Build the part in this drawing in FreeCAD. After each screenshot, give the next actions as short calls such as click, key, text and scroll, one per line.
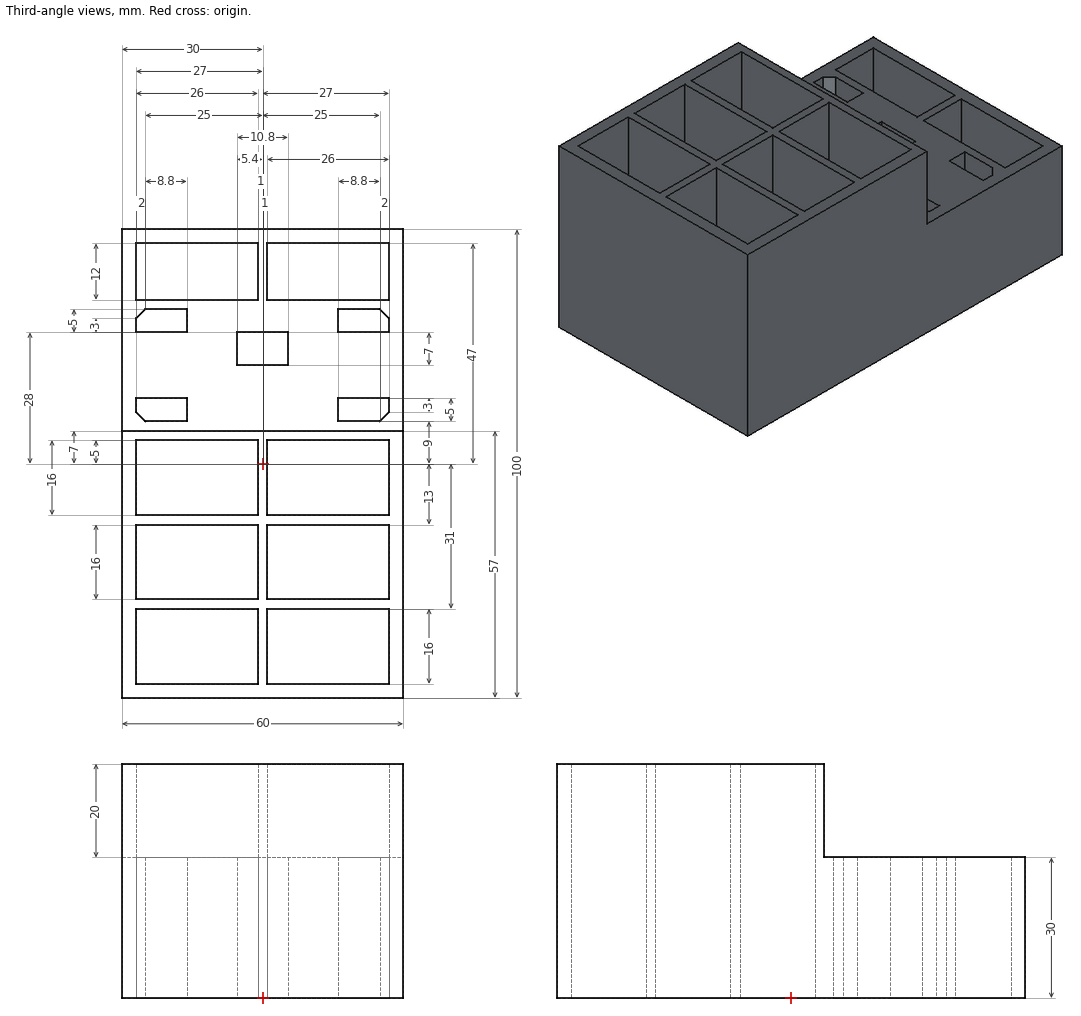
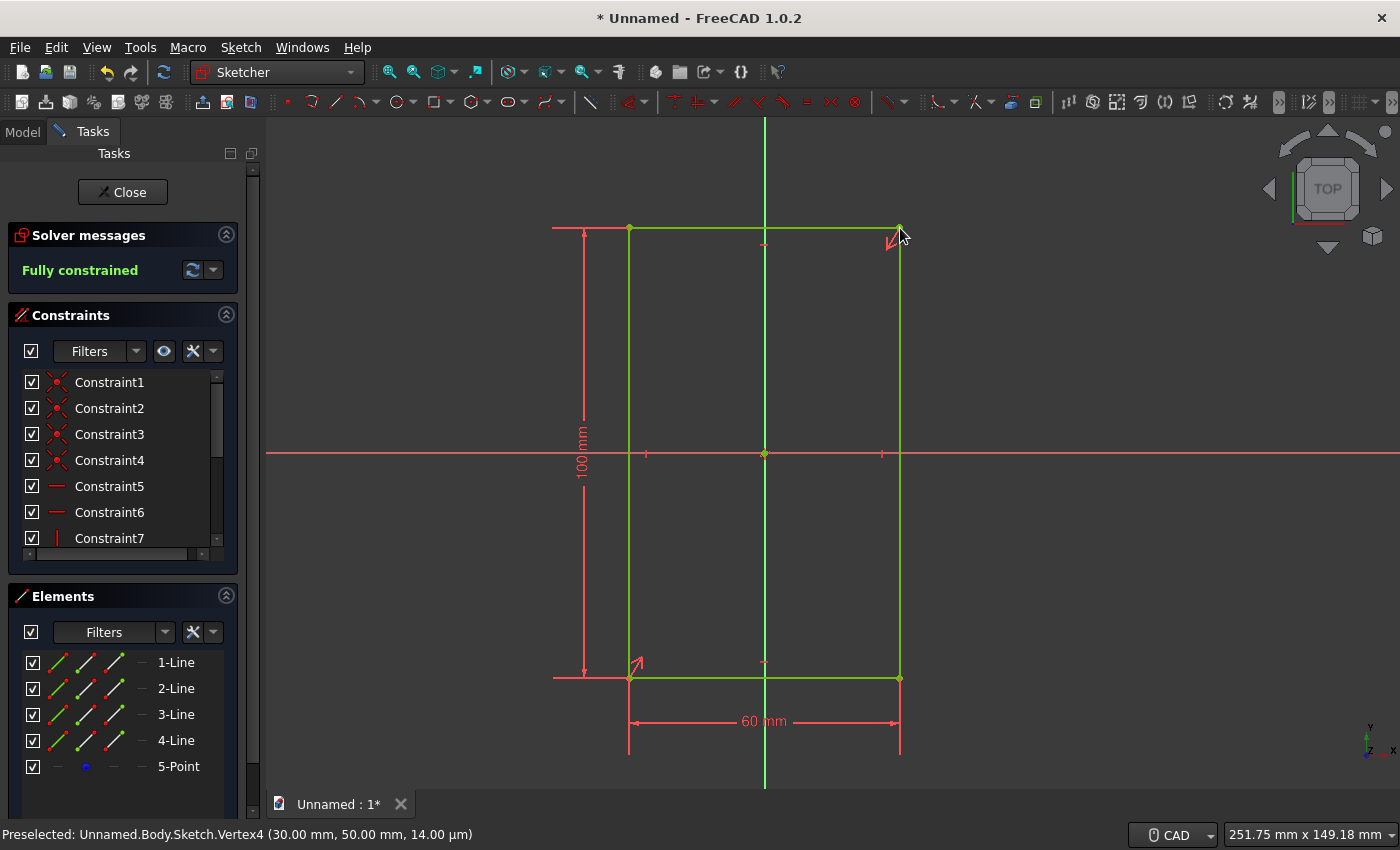
click(123, 192)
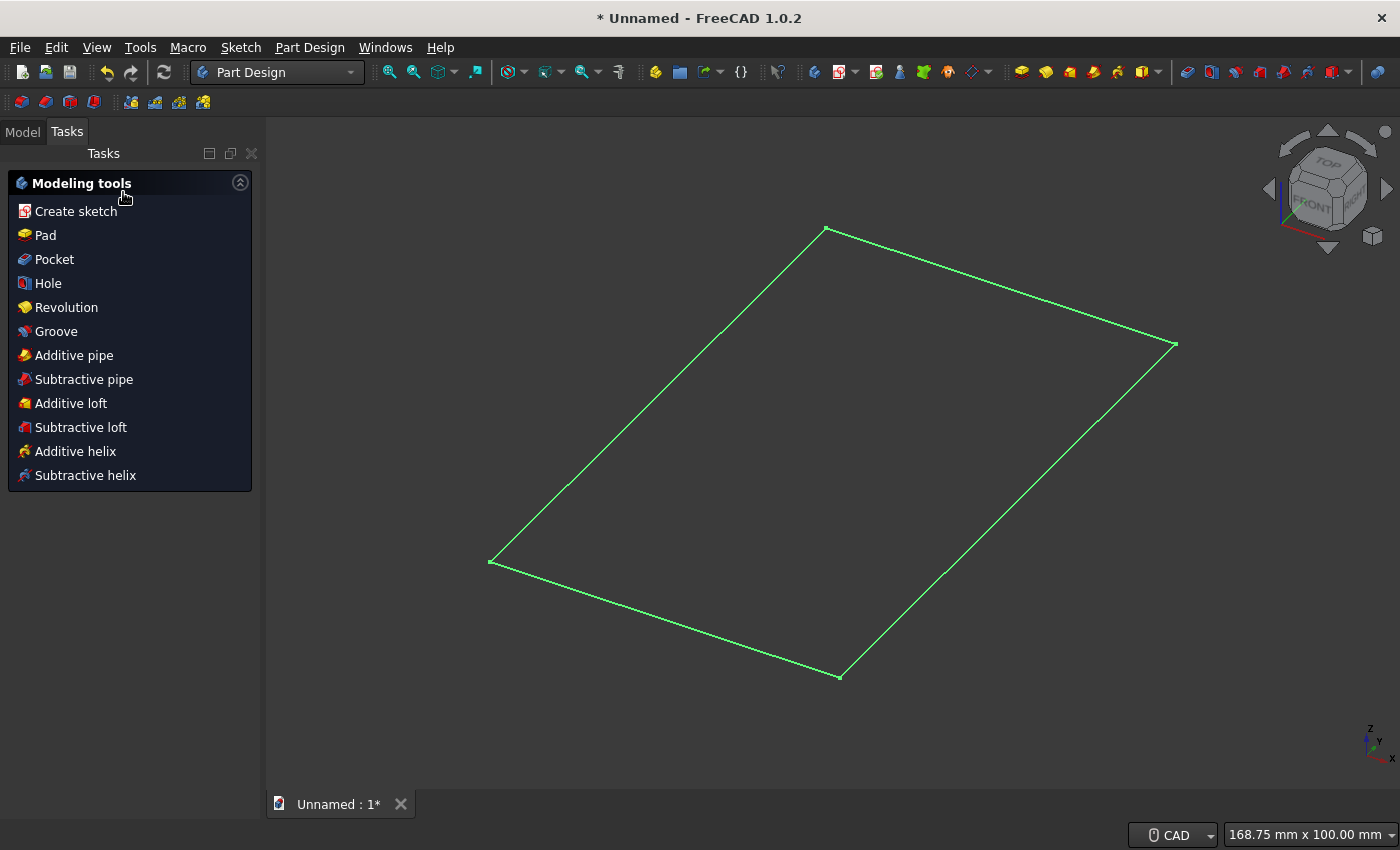
click(1022, 72)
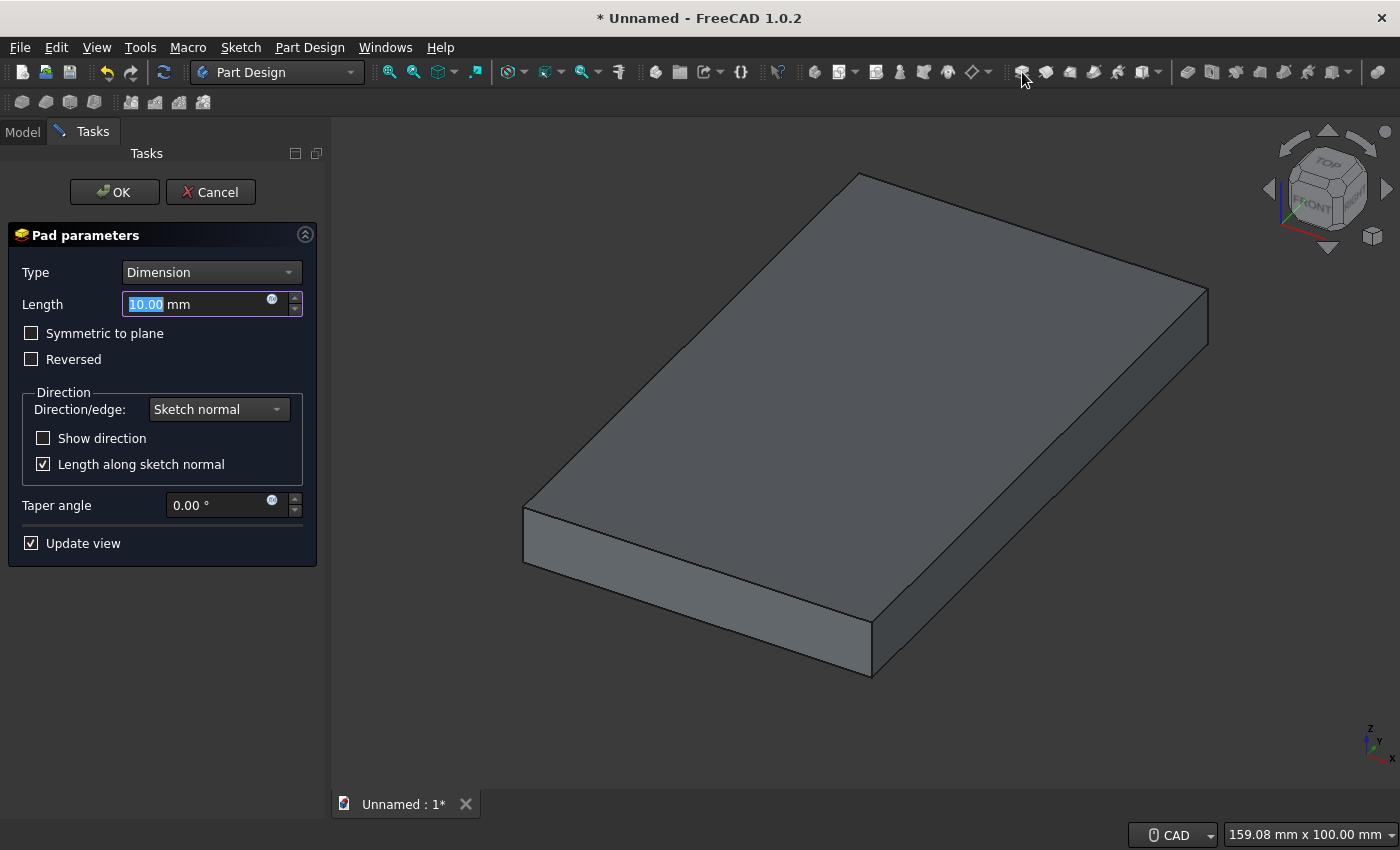
text(30)
key(Tab)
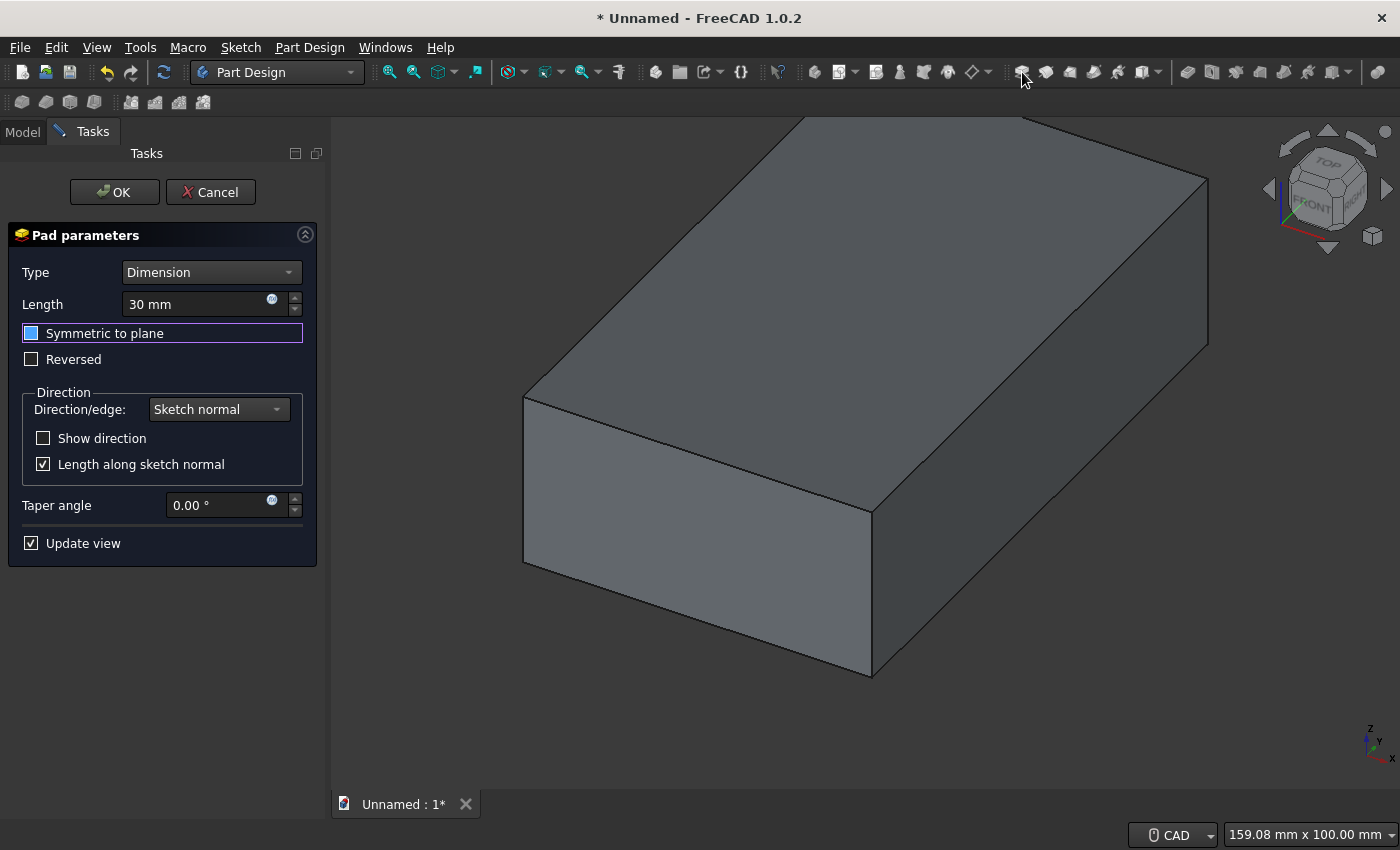
click(115, 192)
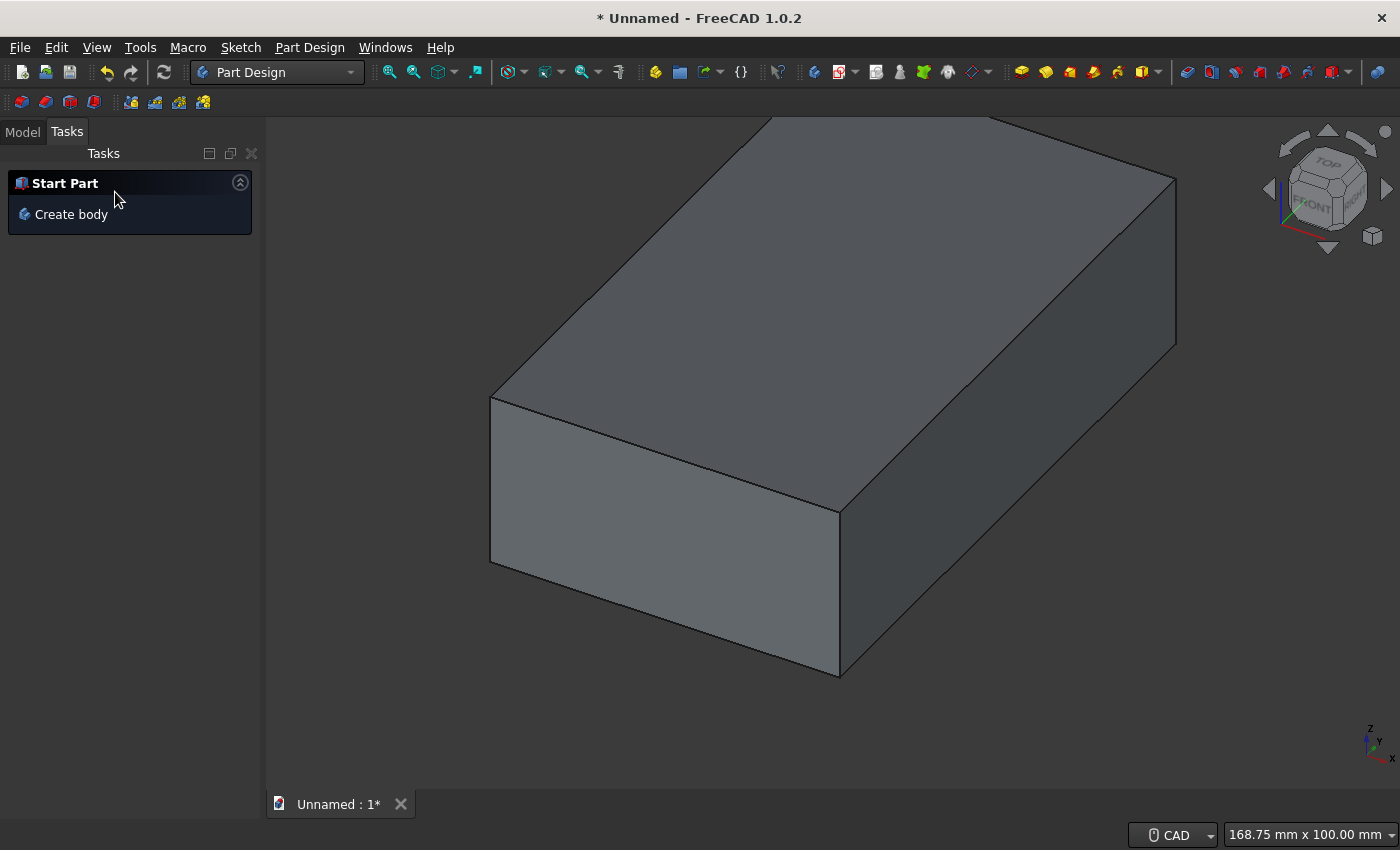
key(v)
key(f)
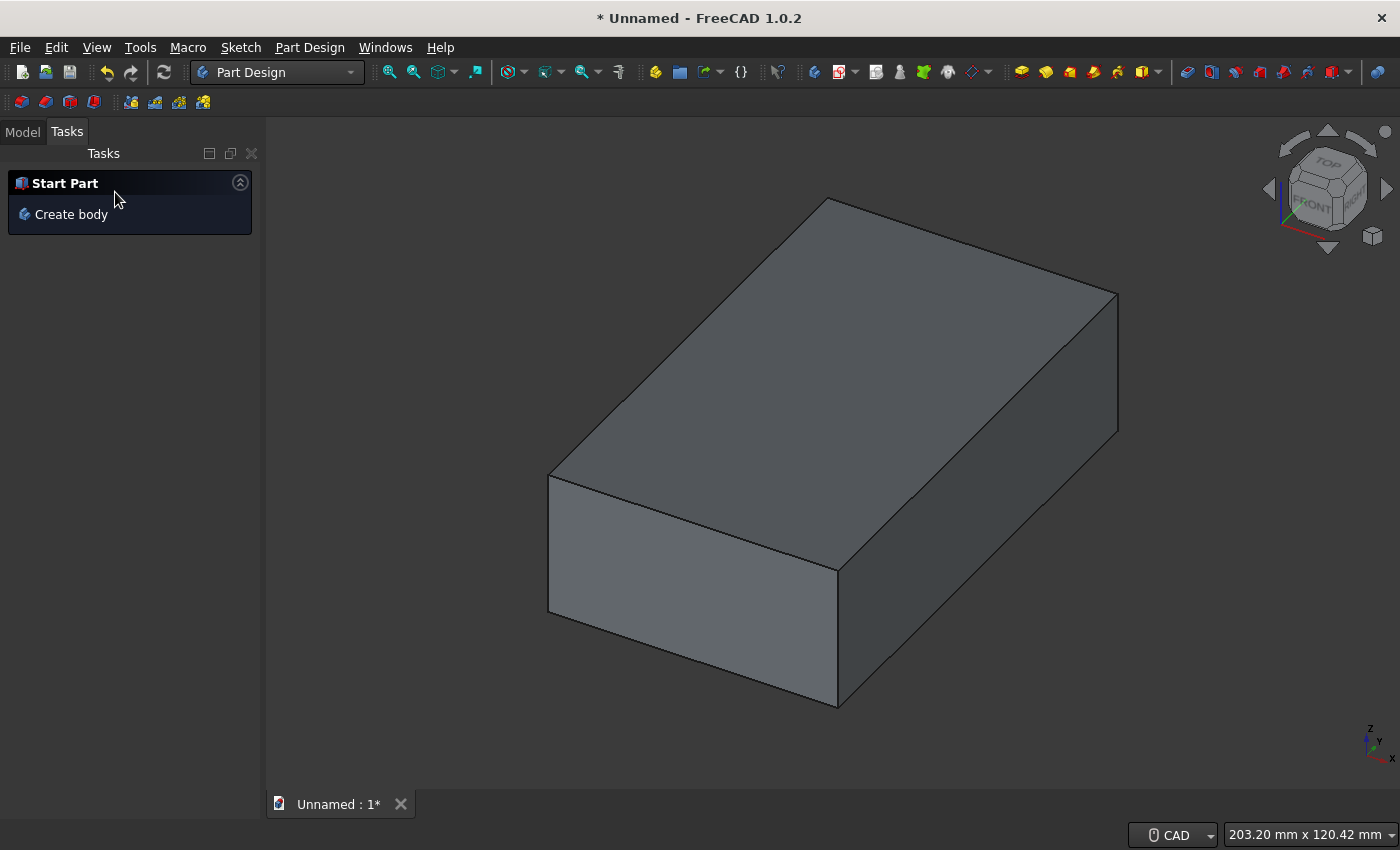
click(873, 344)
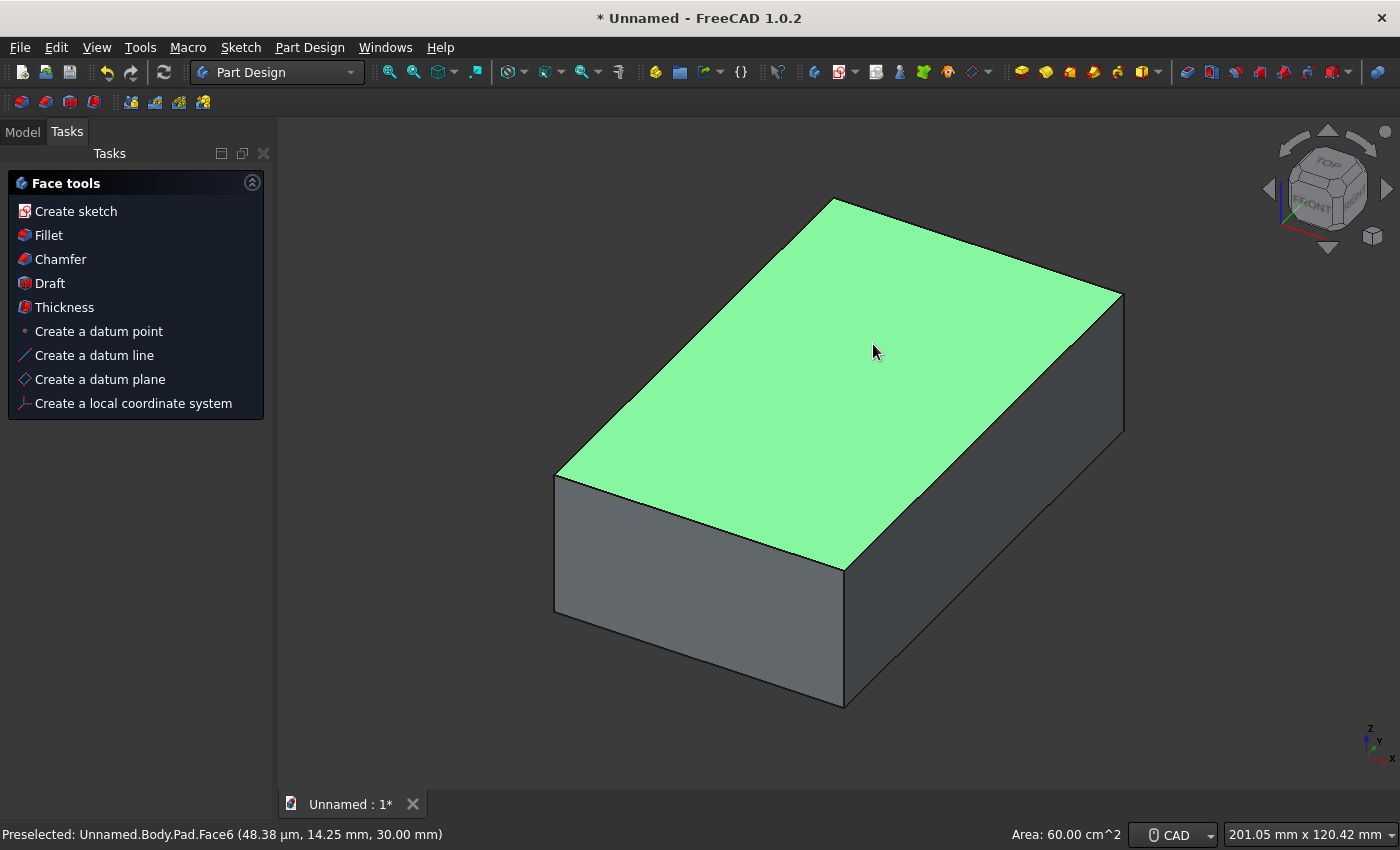
click(840, 72)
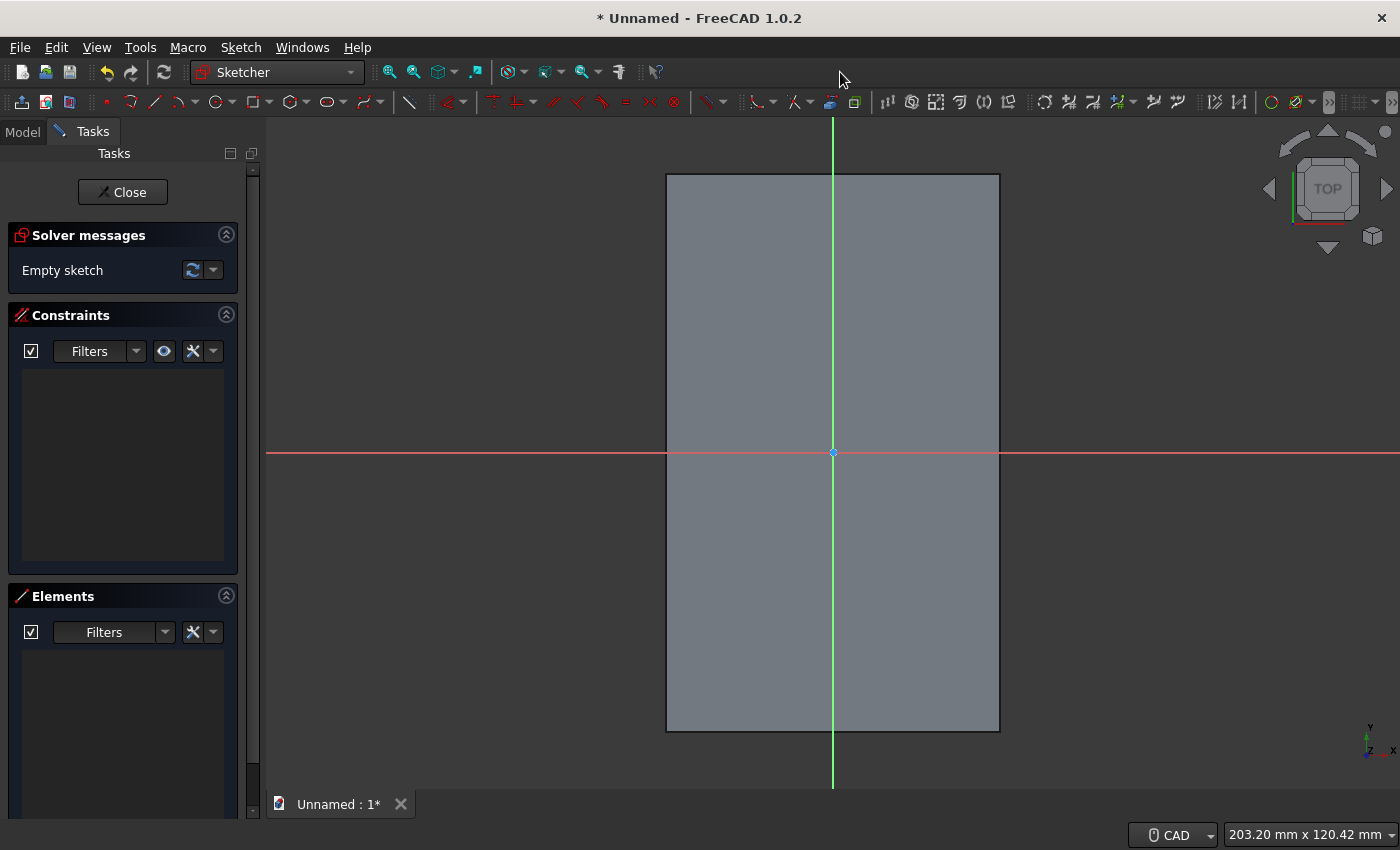
scroll(916, 162, up, 3)